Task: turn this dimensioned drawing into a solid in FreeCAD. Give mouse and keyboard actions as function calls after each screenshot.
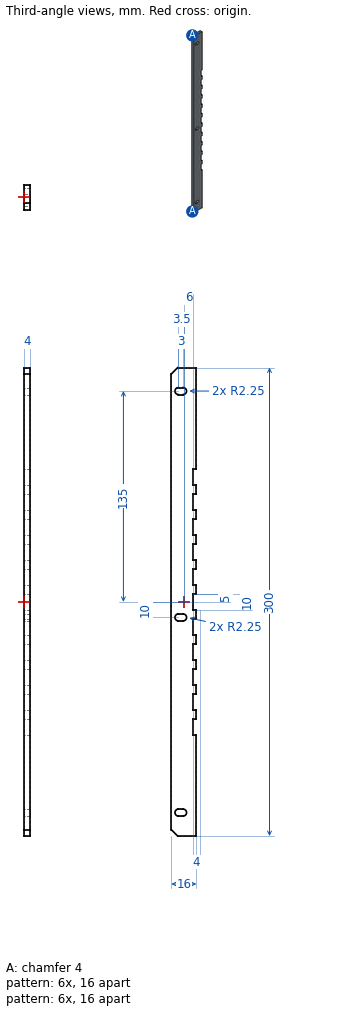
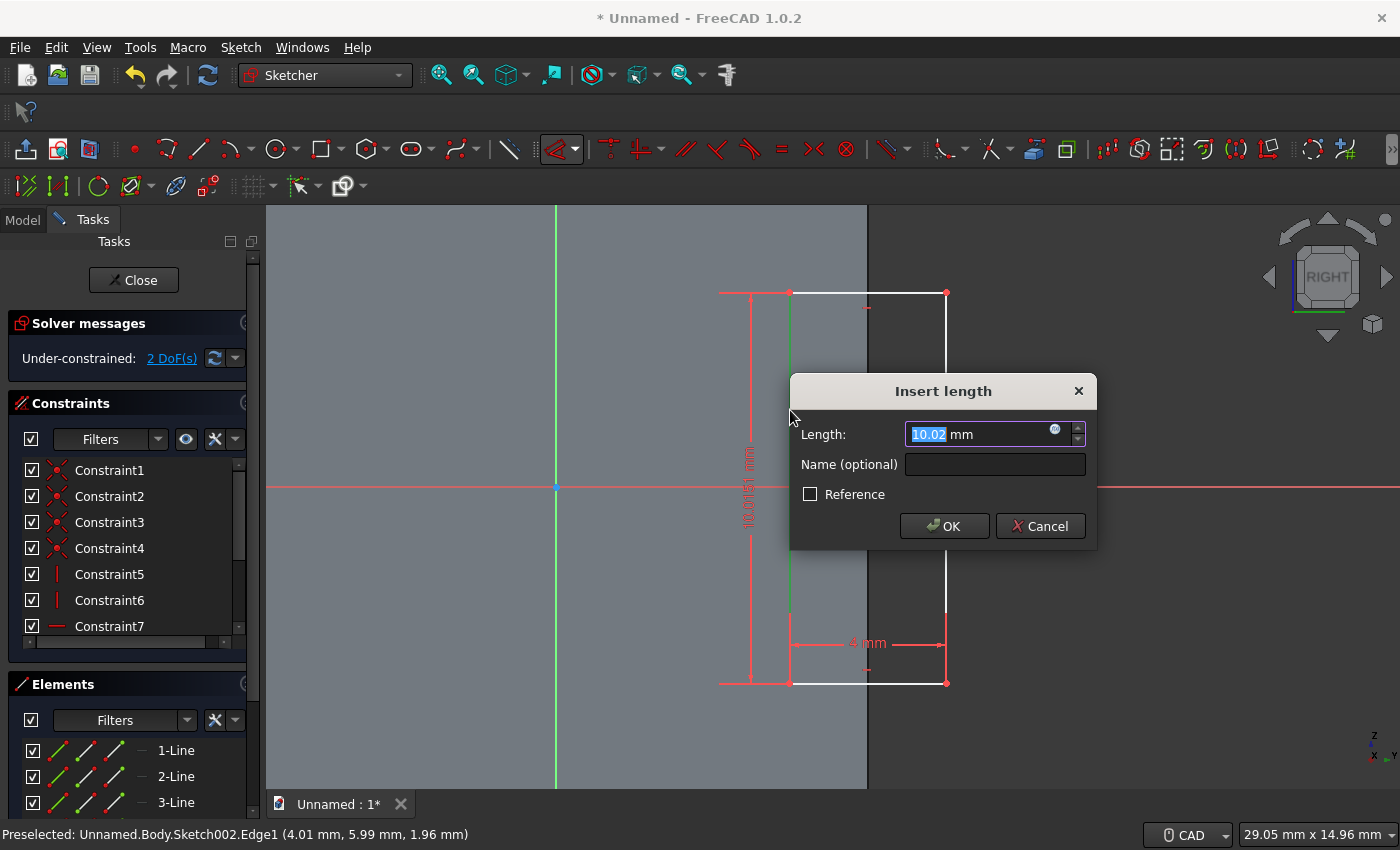
text(10)
key(Return)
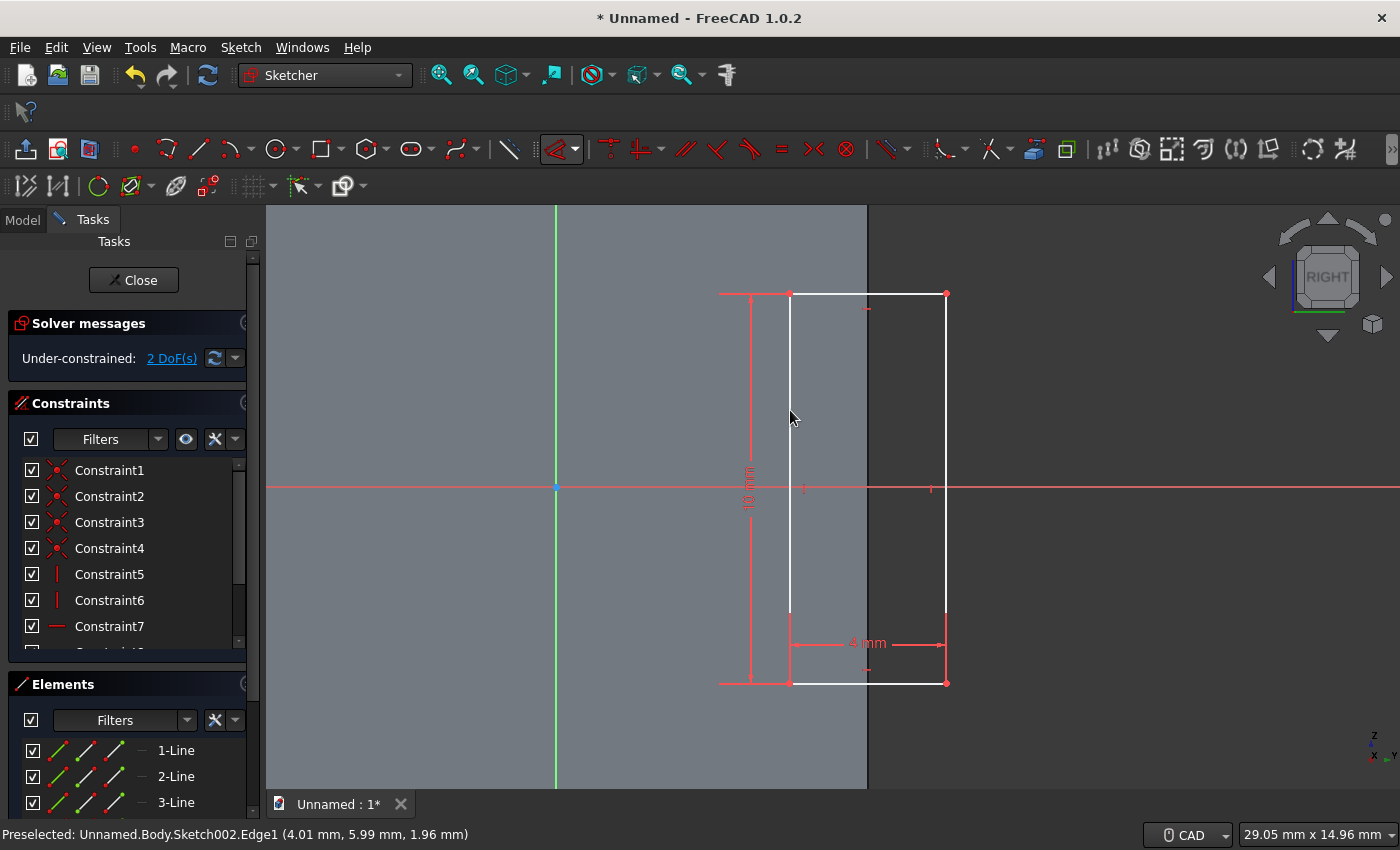
click(790, 294)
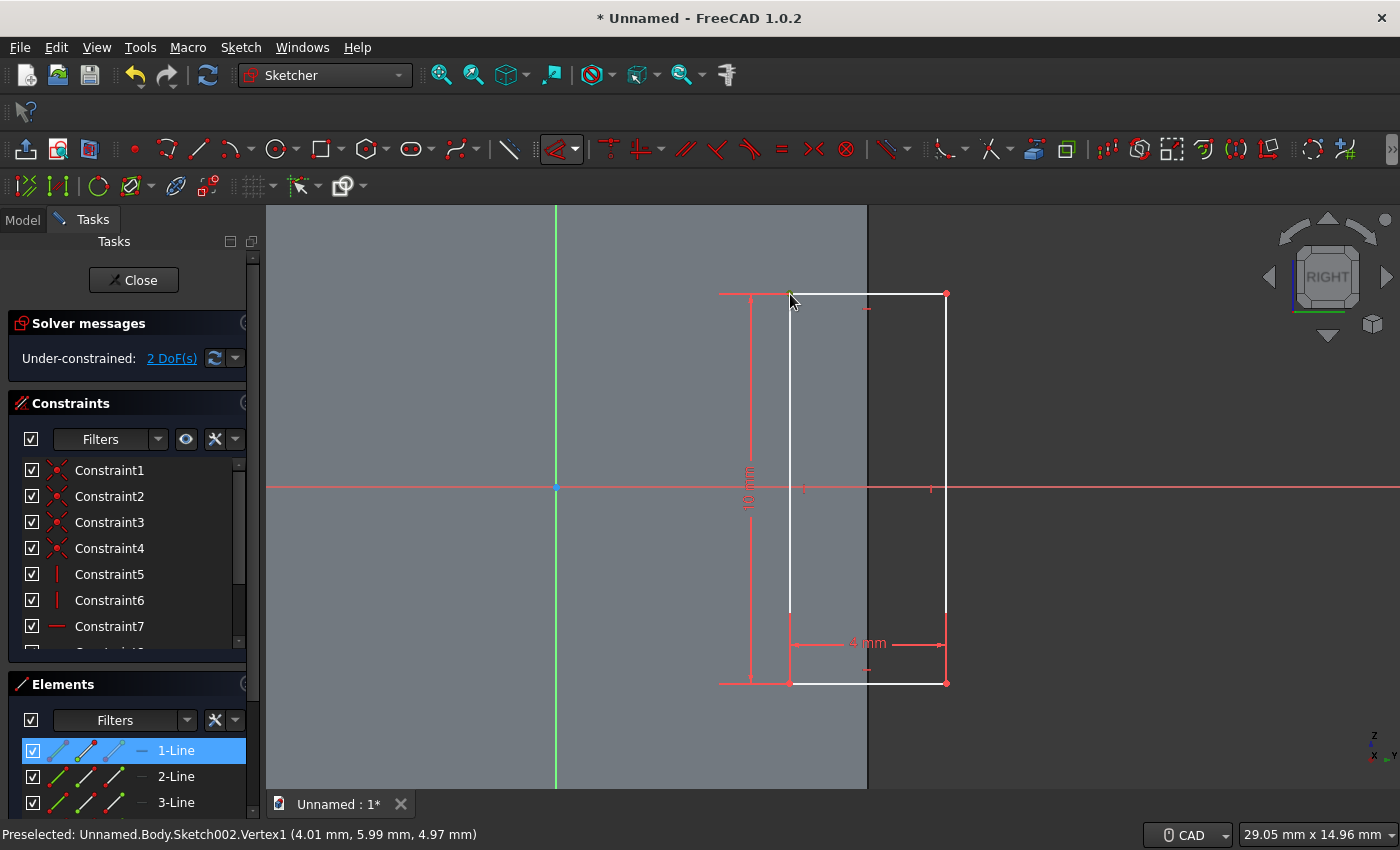
key(l)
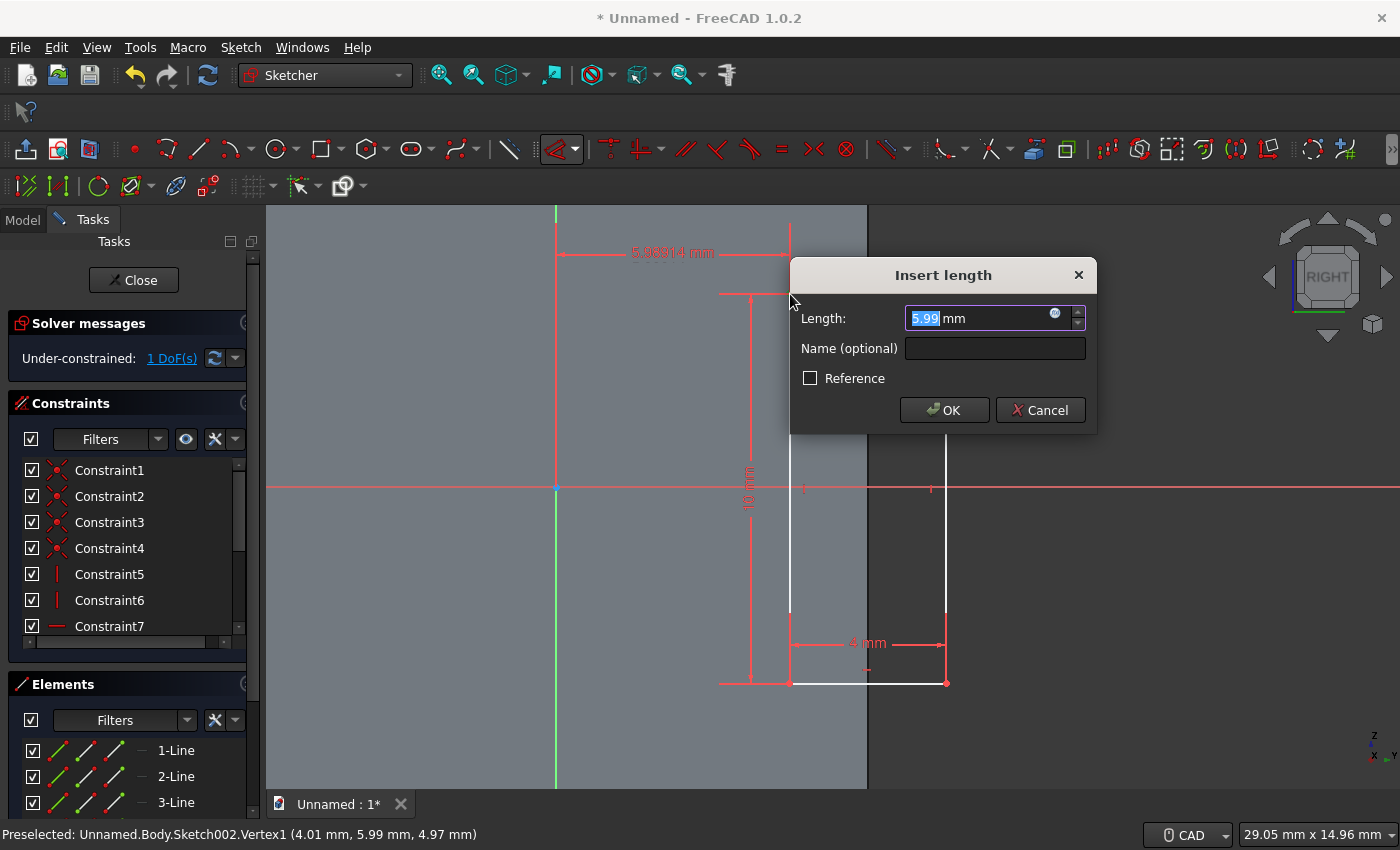
text(6)
key(Return)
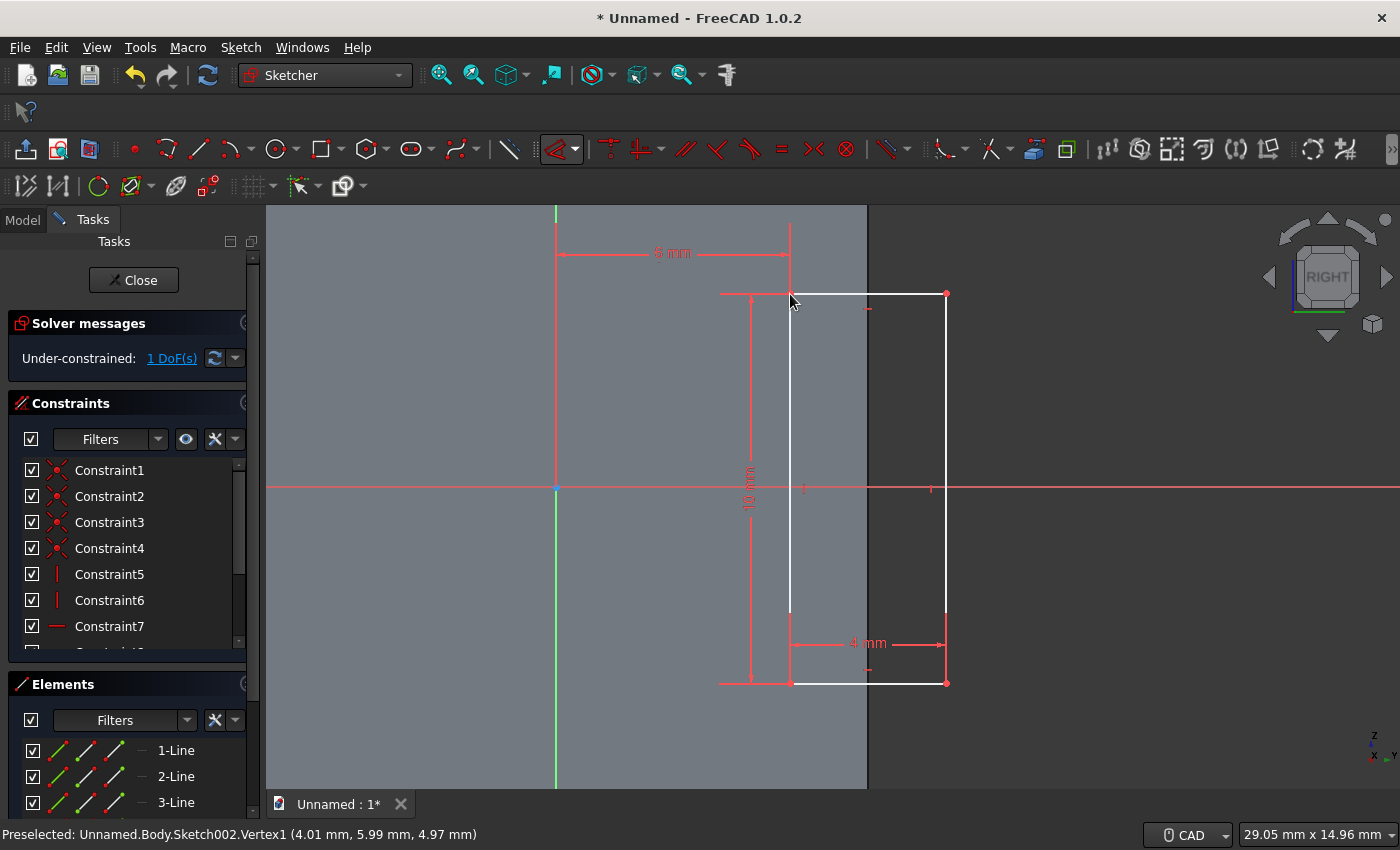
click(790, 294)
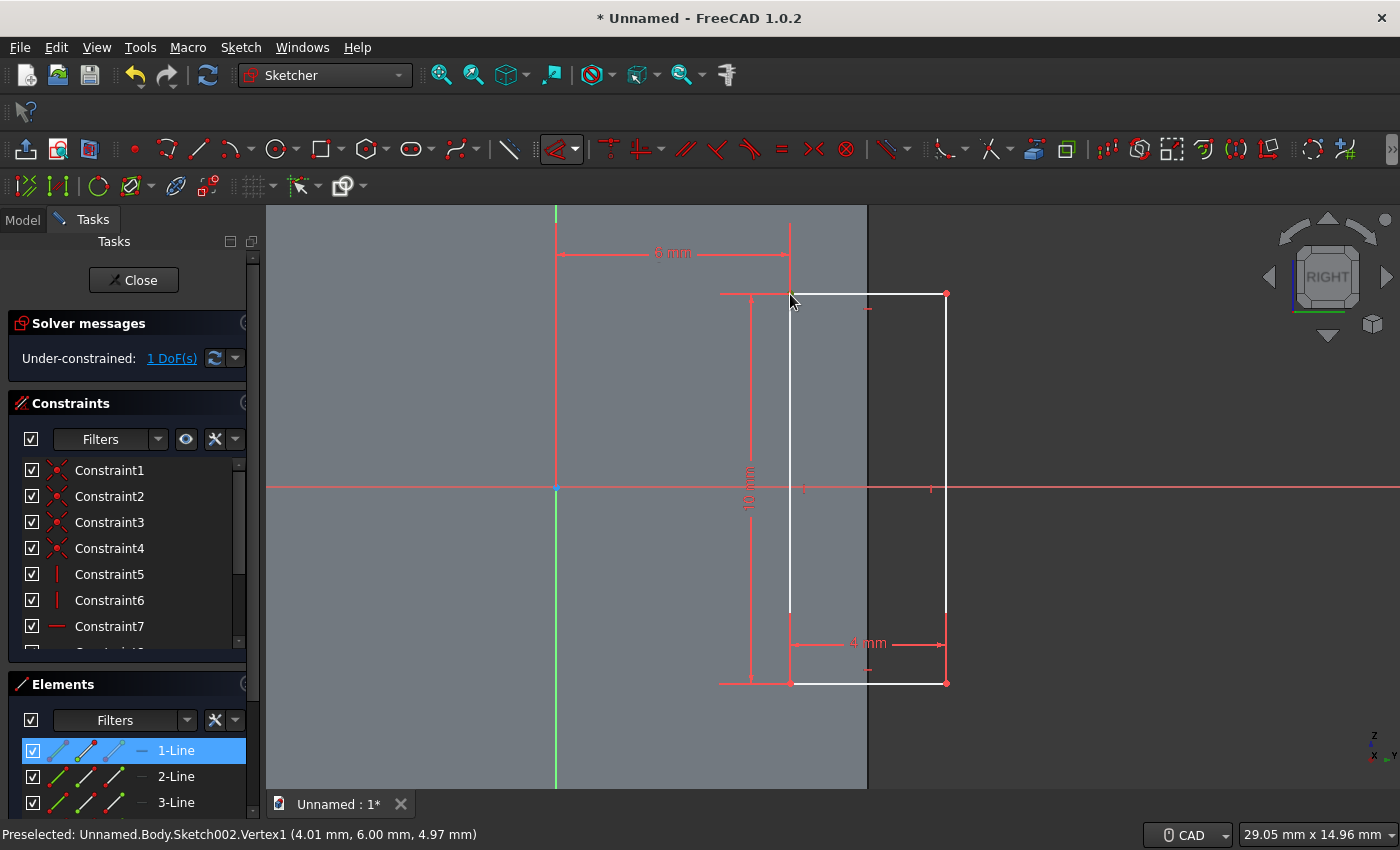
key(i)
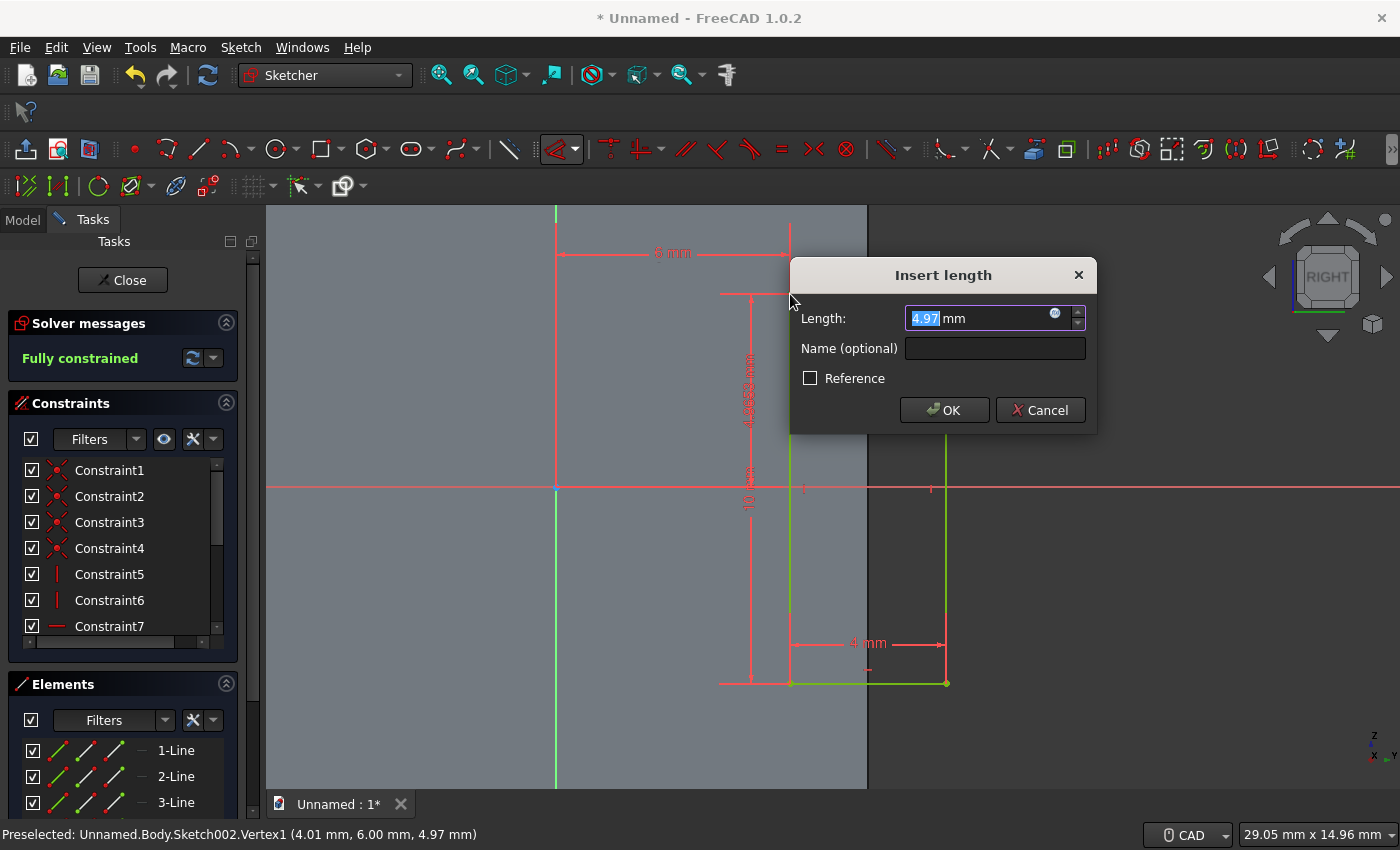
text(5)
key(Return)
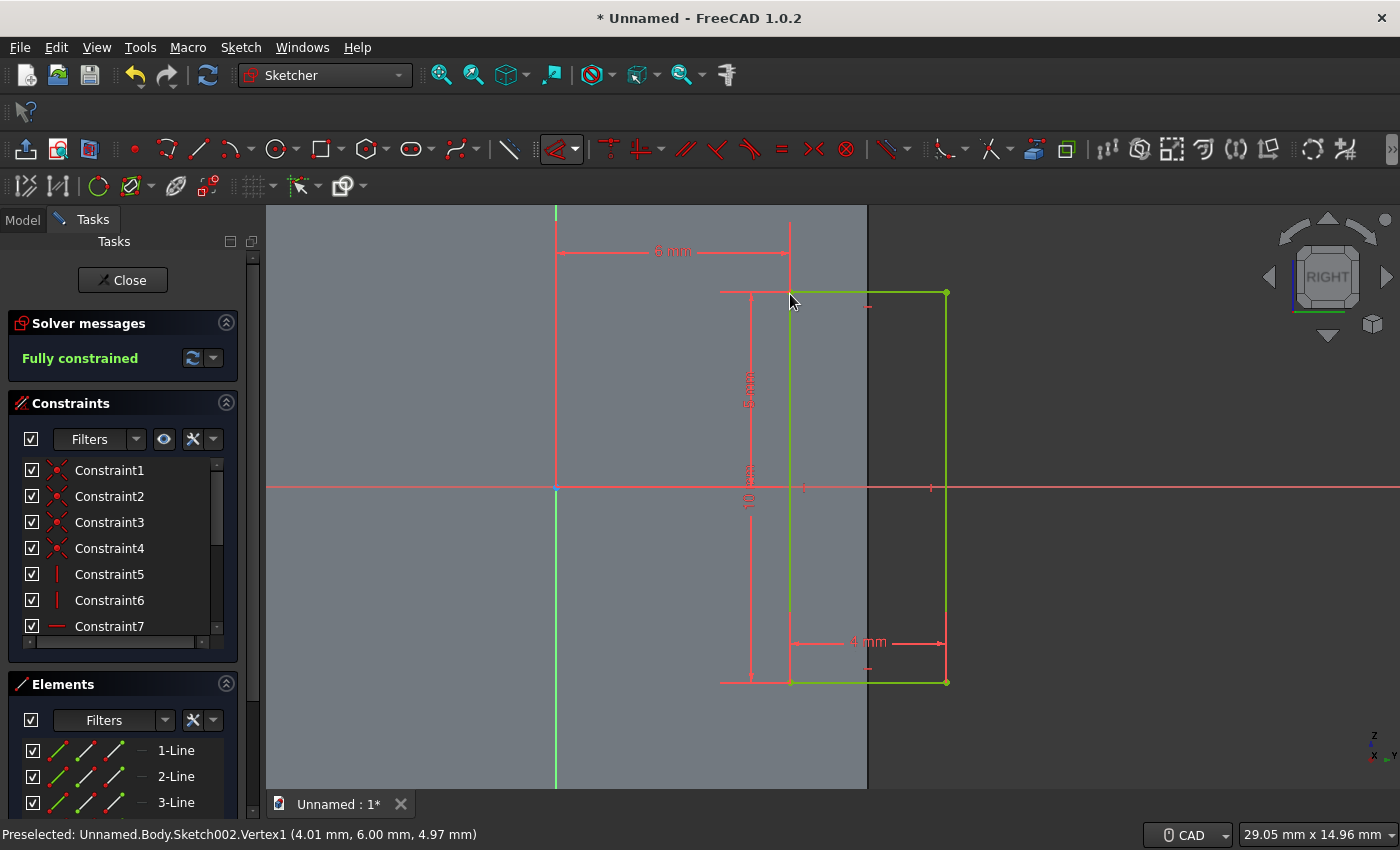
click(123, 280)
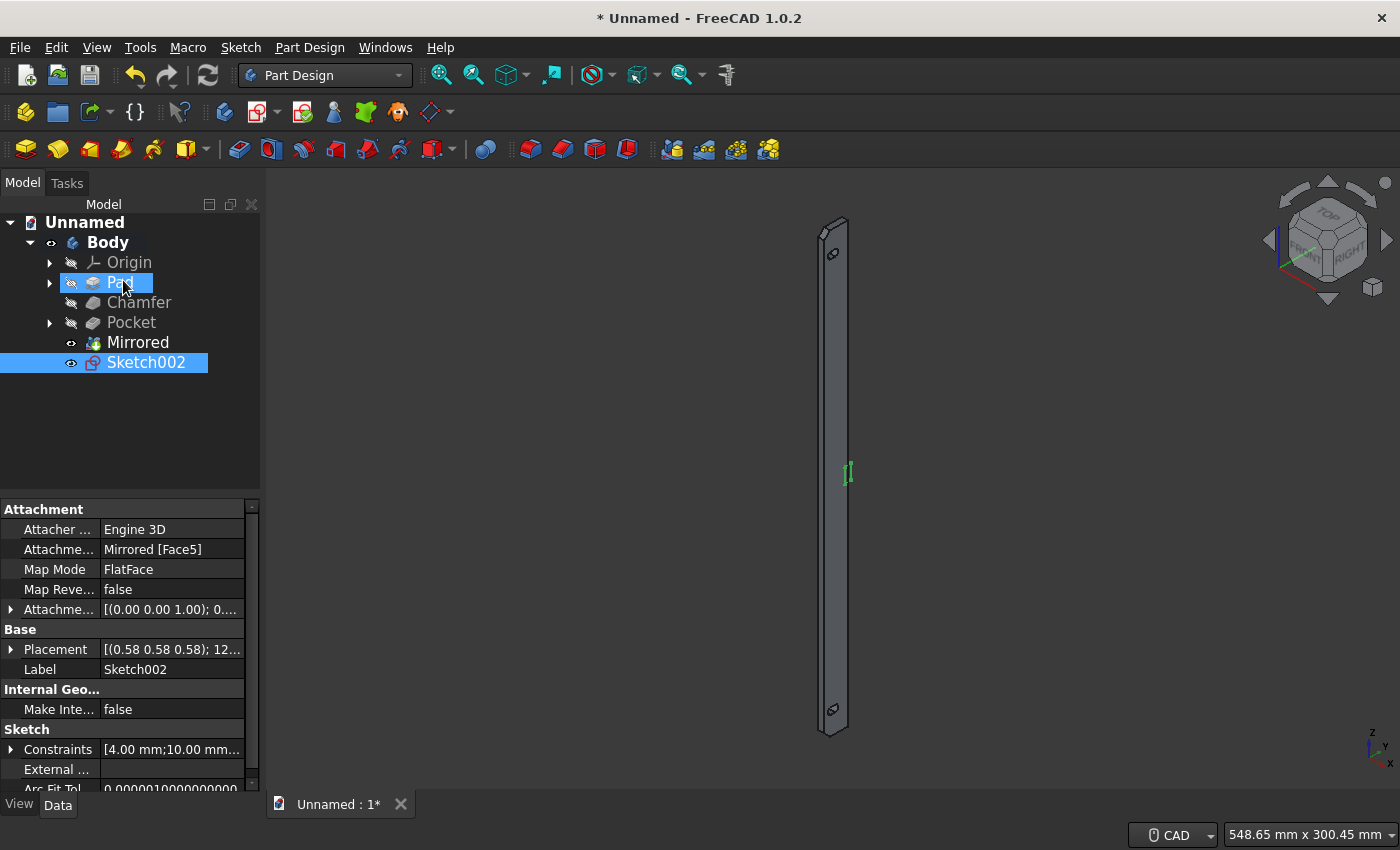
click(240, 150)